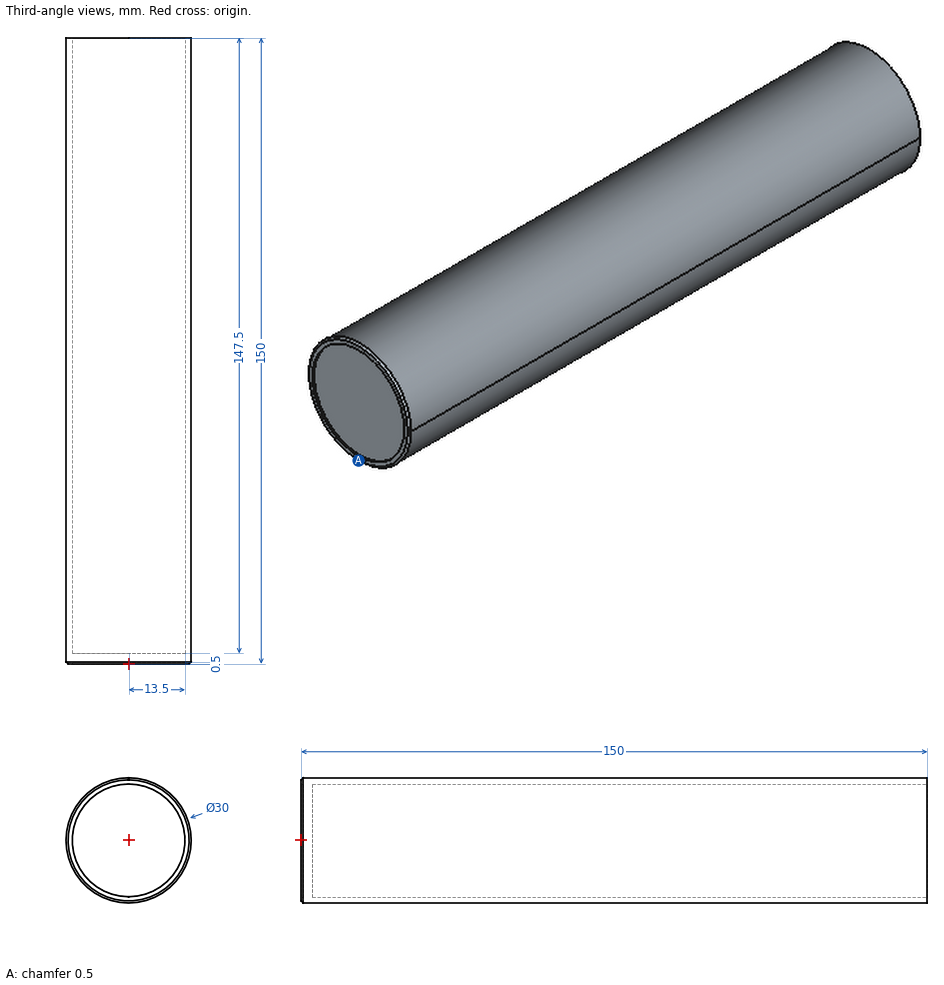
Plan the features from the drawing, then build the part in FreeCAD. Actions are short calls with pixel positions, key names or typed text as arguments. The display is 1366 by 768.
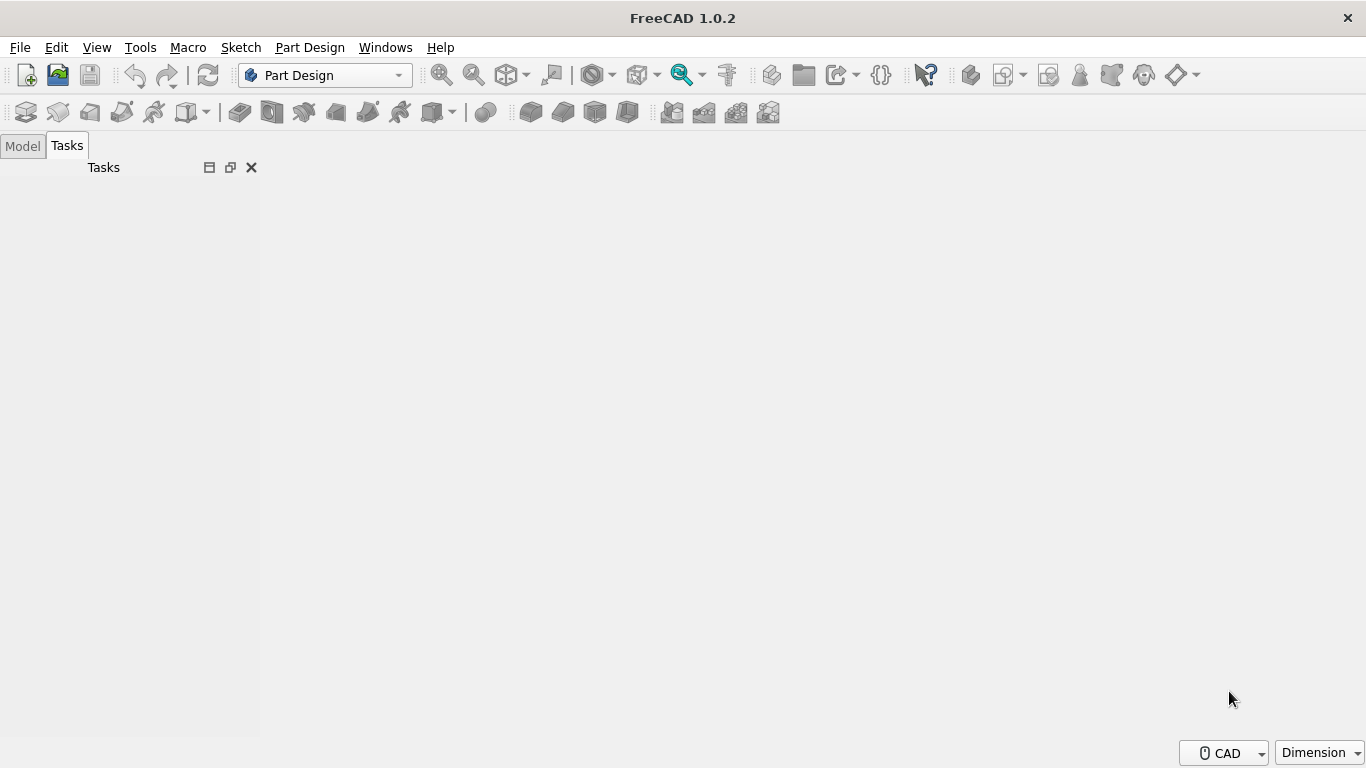
click(26, 76)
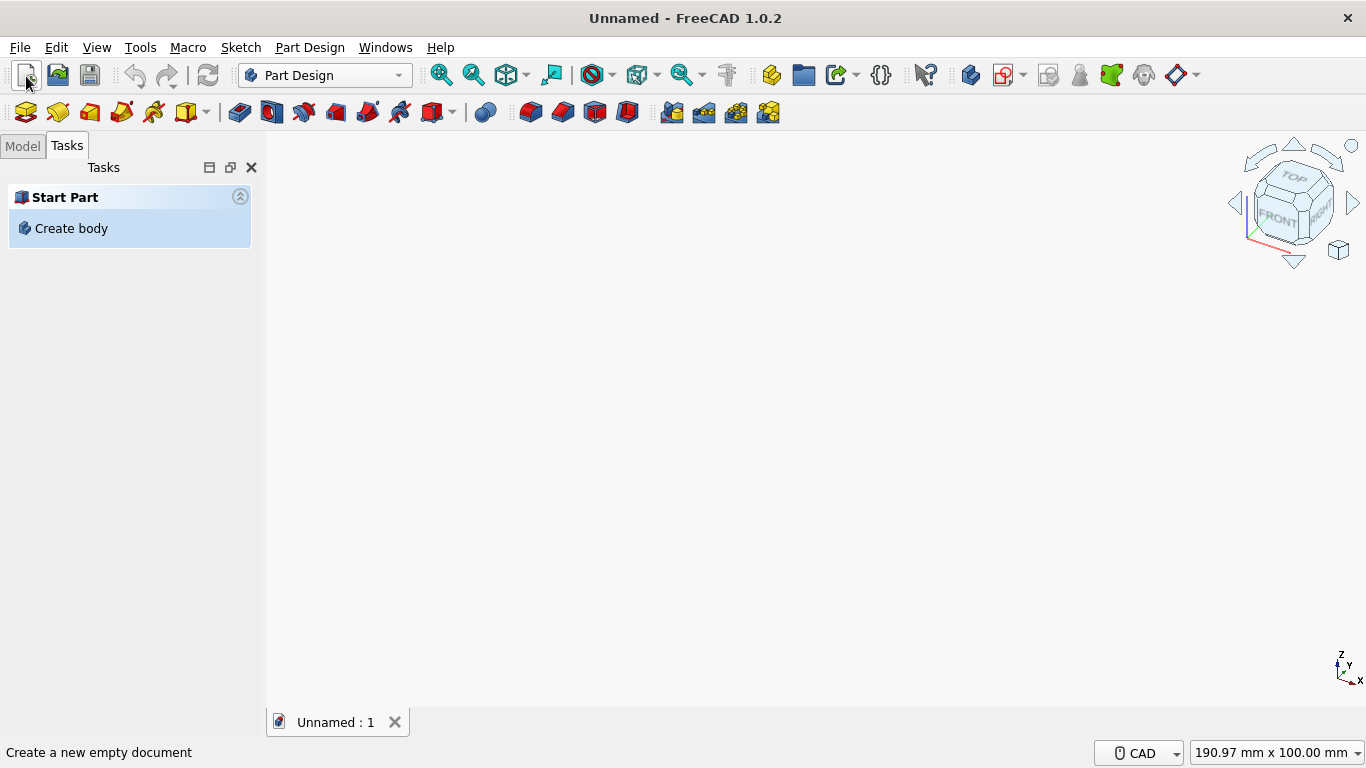
click(1004, 76)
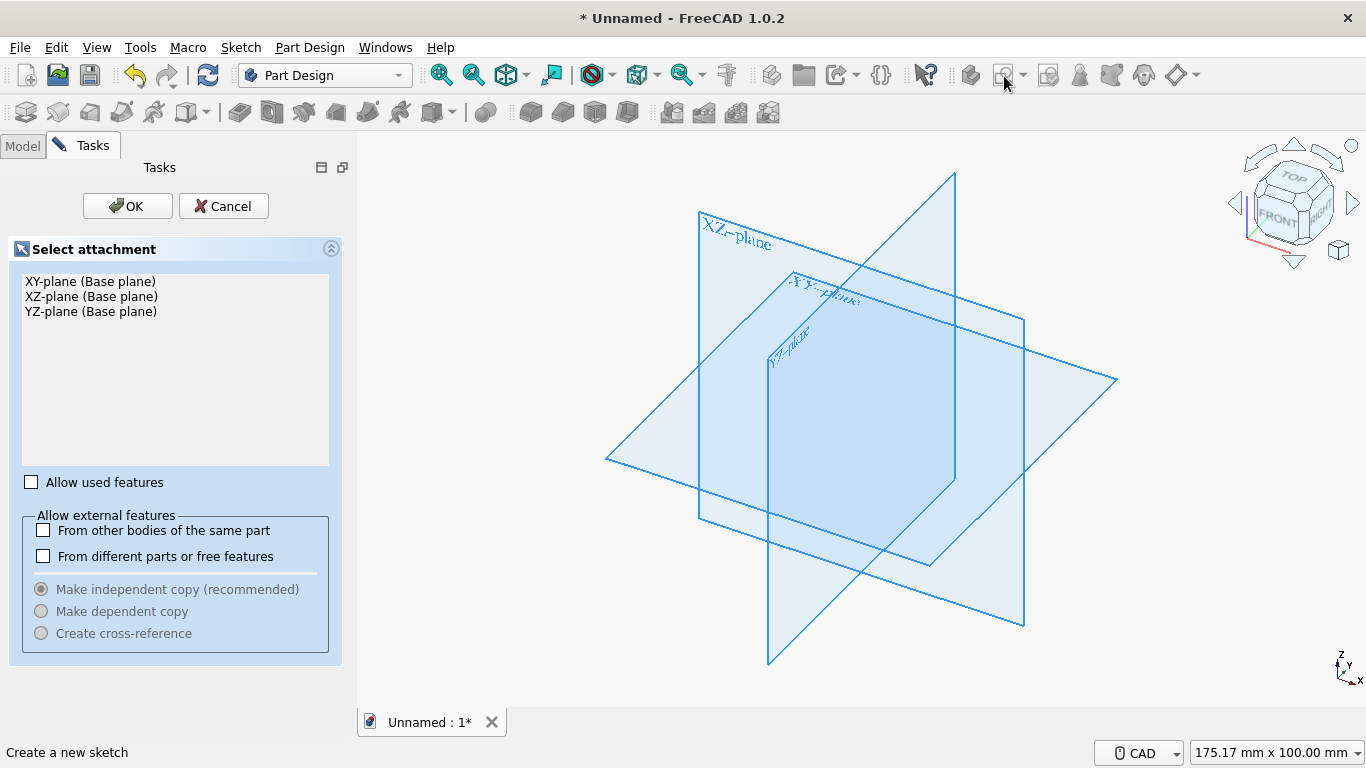
click(82, 296)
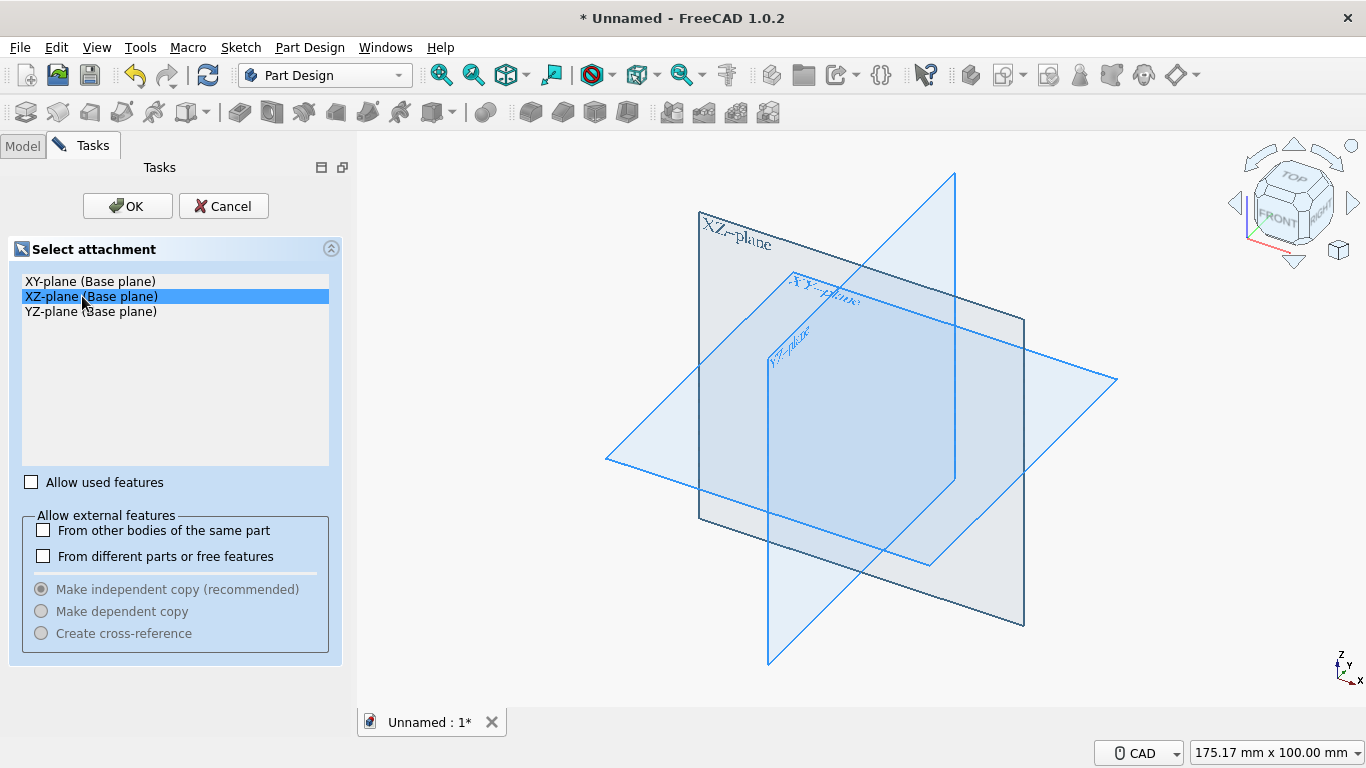
click(128, 206)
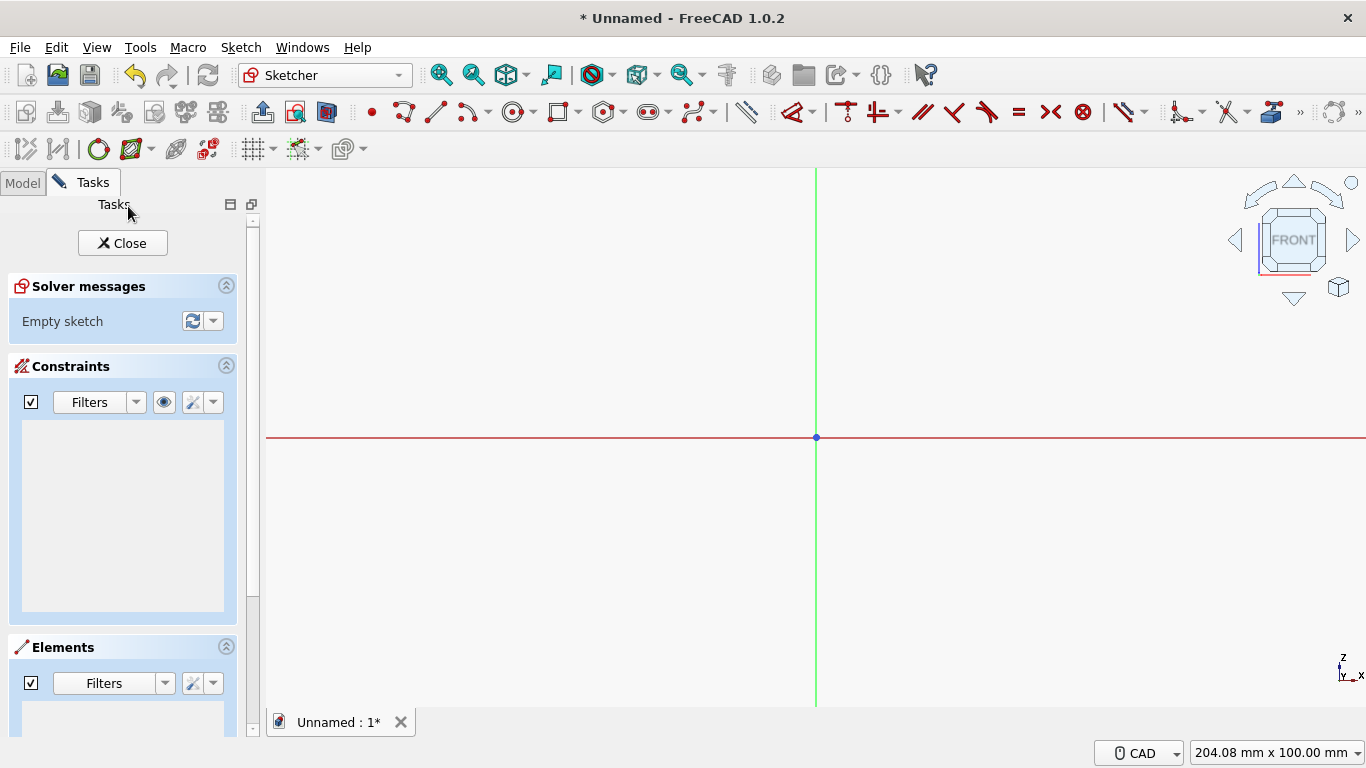
scroll(872, 438, up, 4)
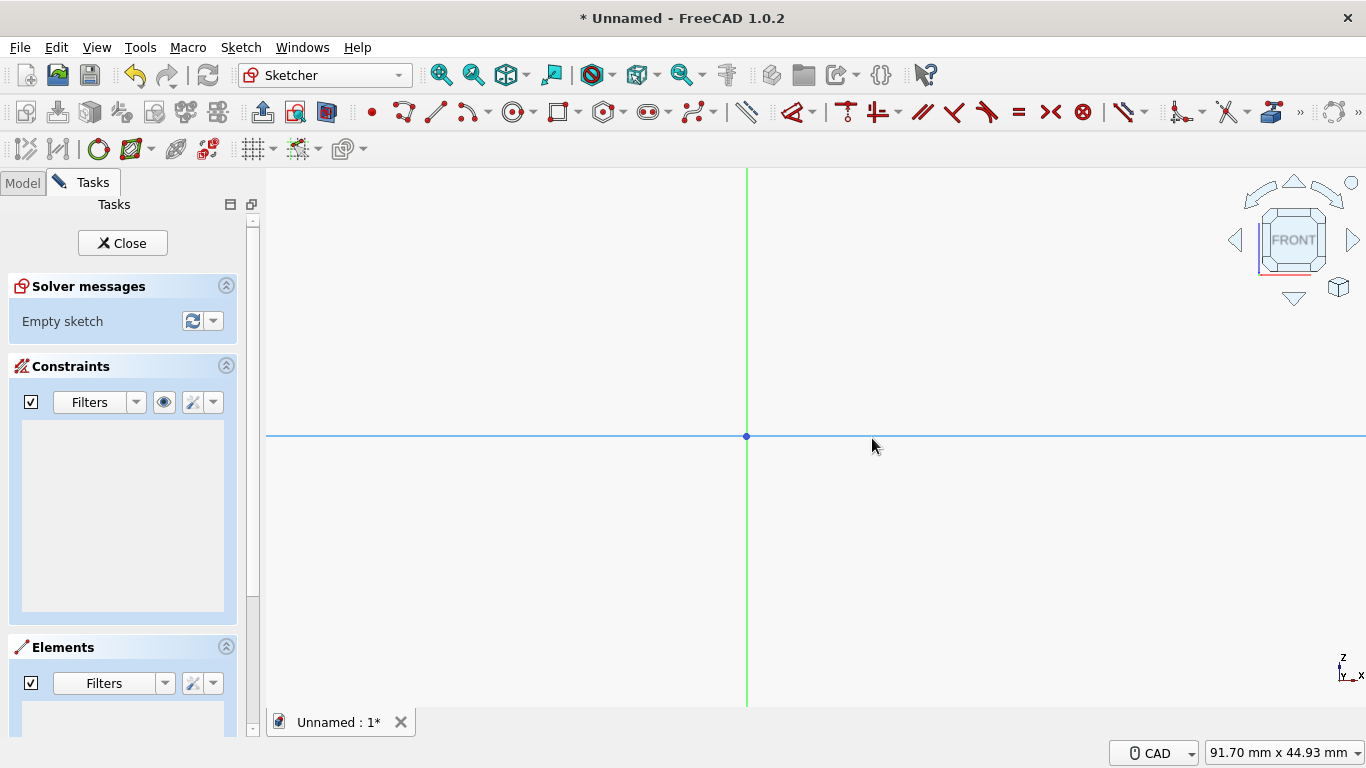
click(514, 112)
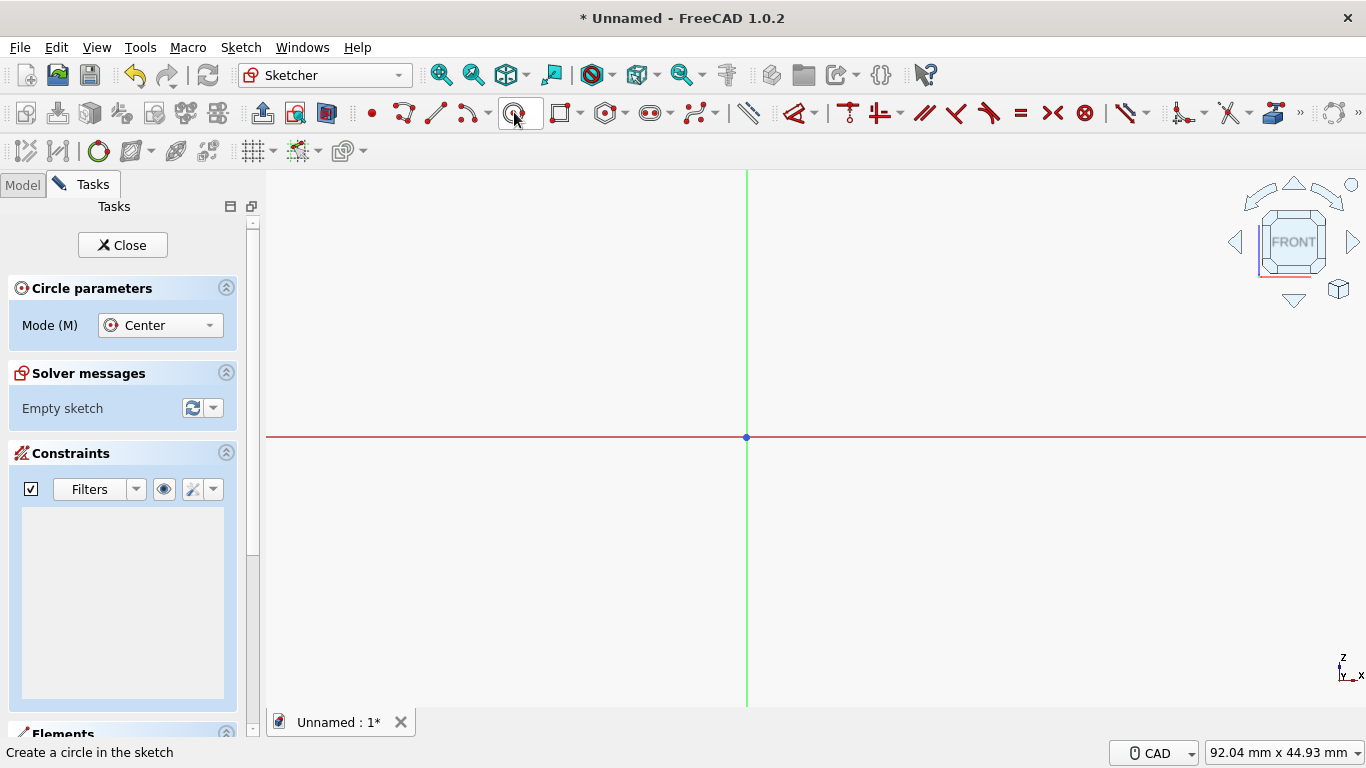
click(747, 437)
move(874, 311)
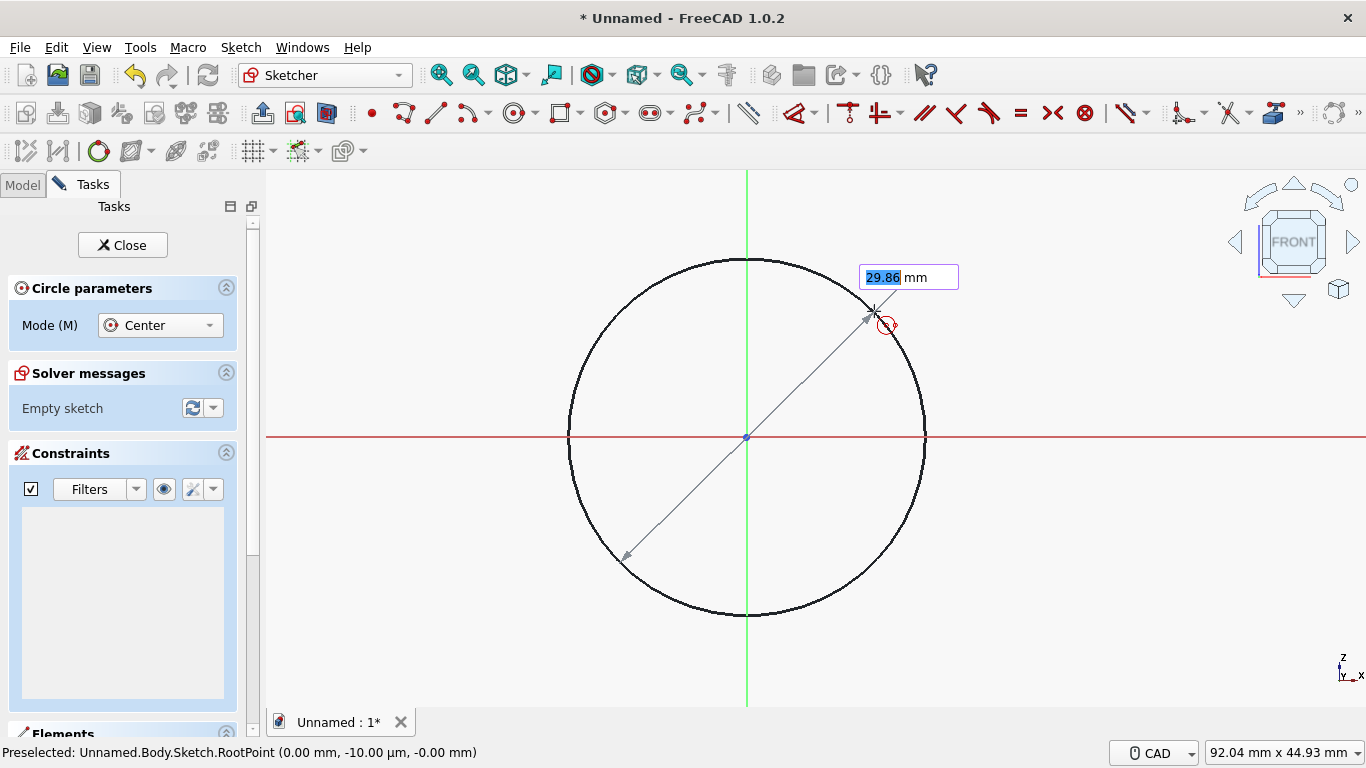
text(30)
key(Return)
key(Escape)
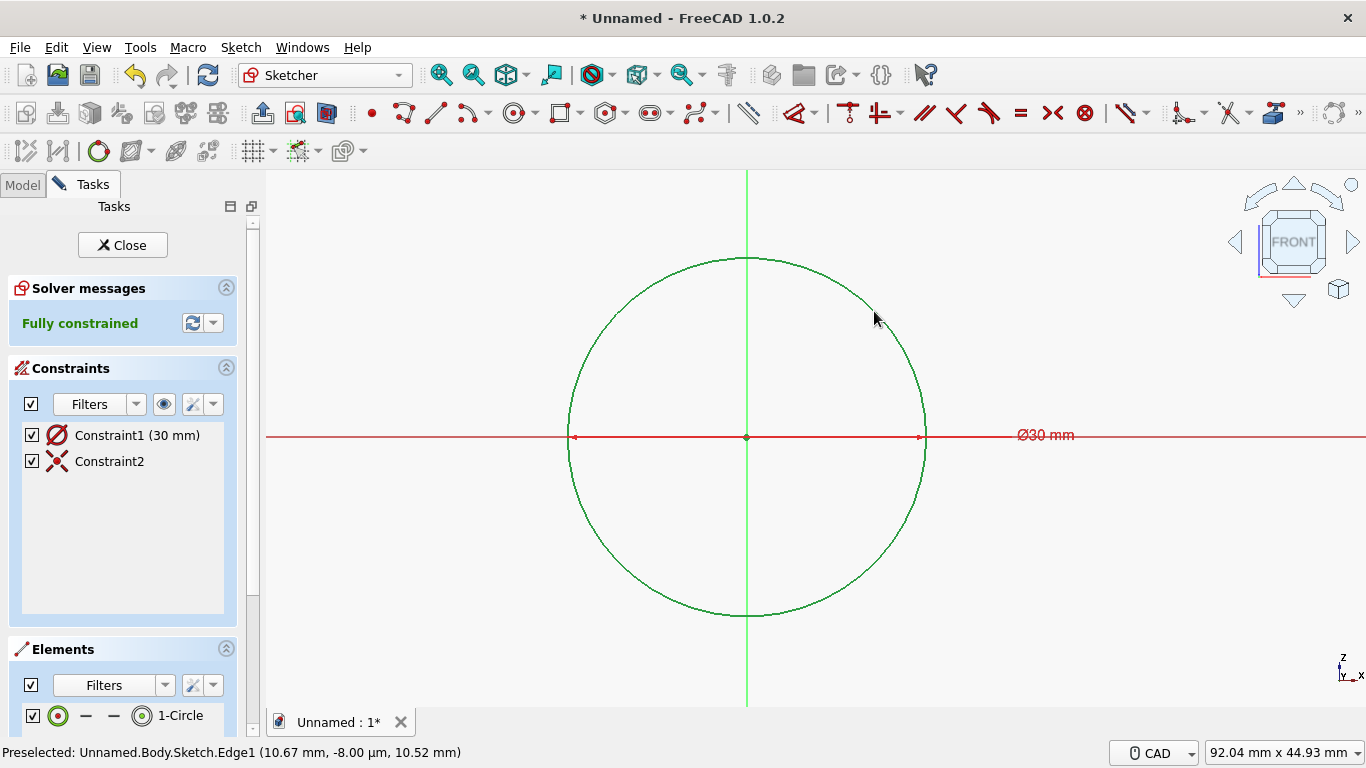
click(123, 245)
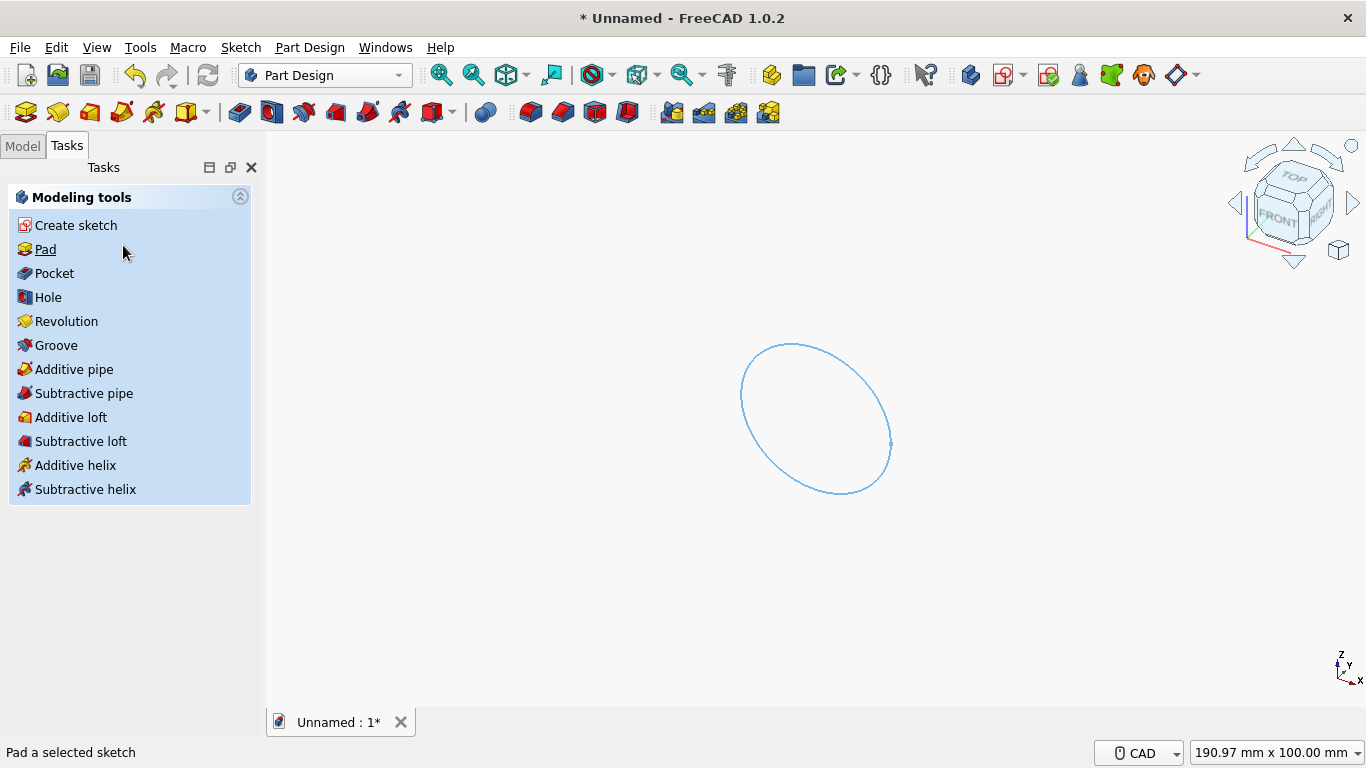
click(26, 112)